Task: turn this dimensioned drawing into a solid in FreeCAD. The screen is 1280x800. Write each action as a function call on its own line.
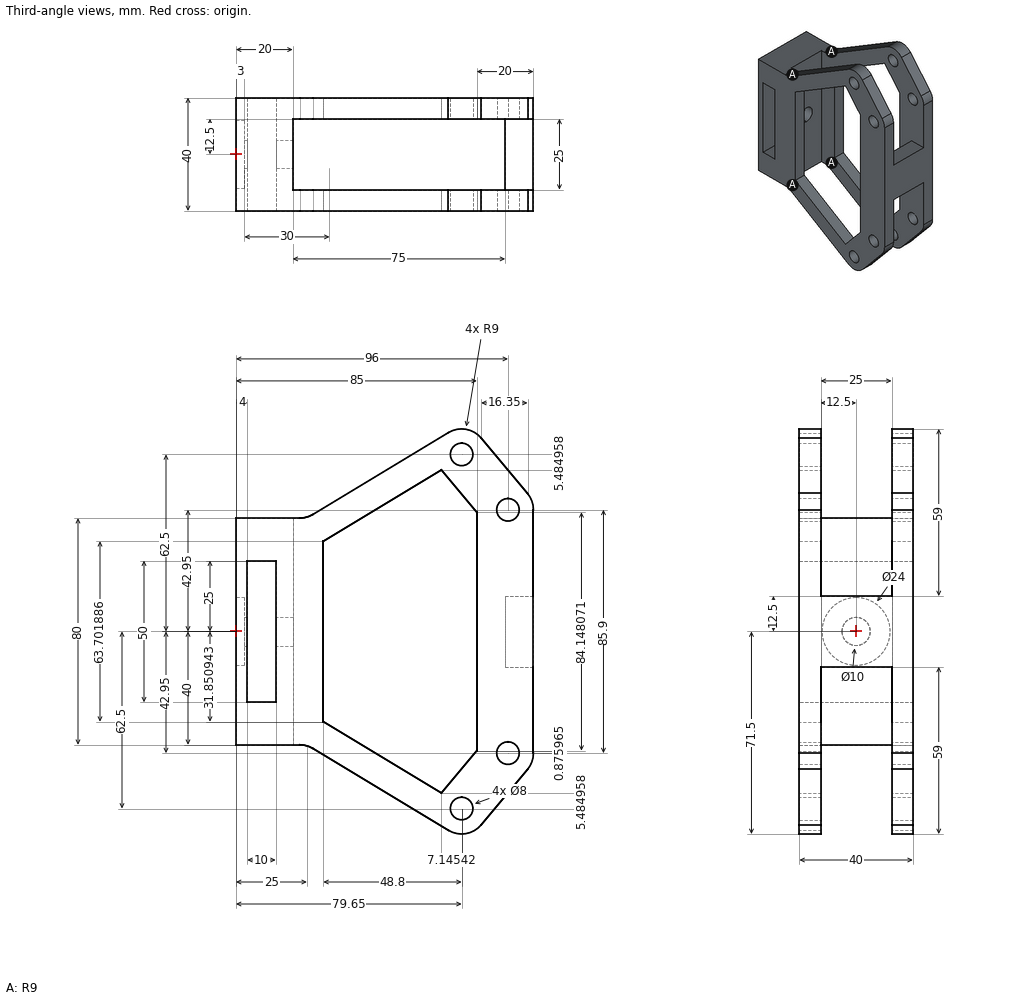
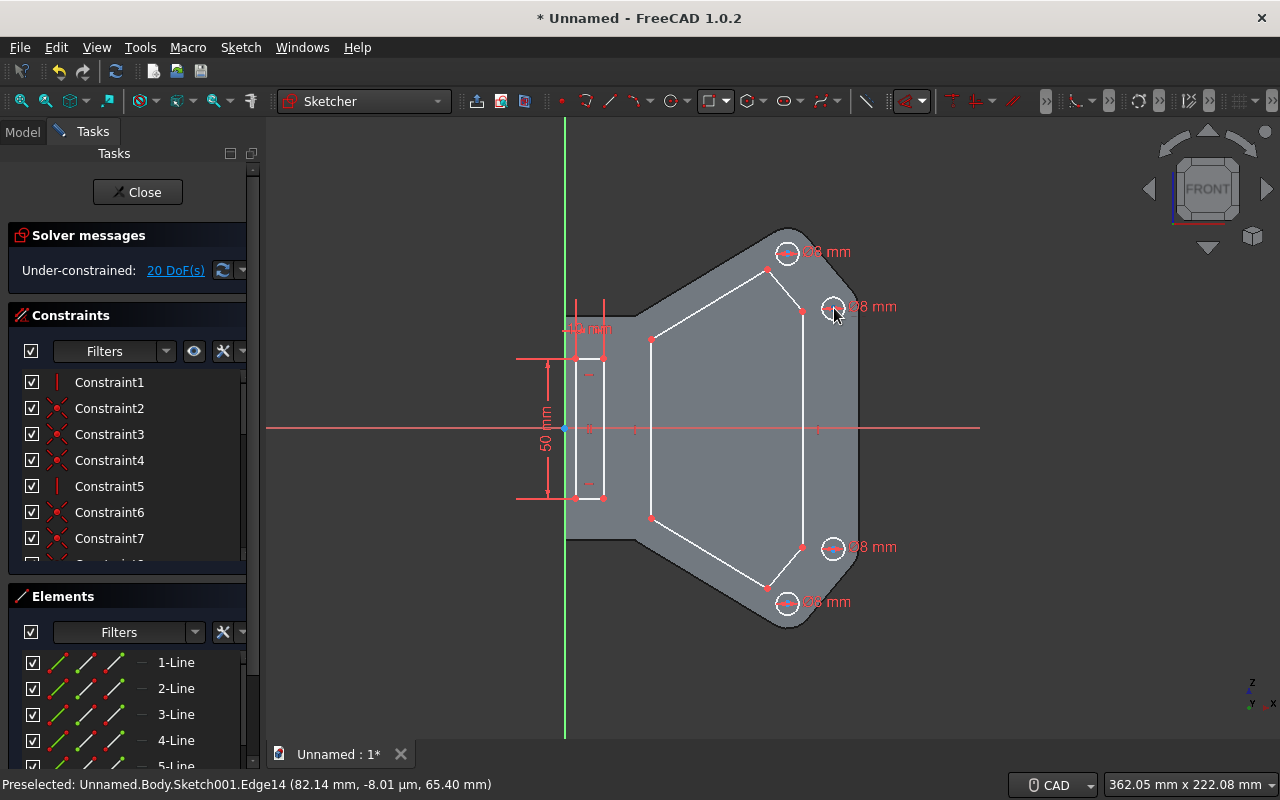
scroll(576, 359, up, 7)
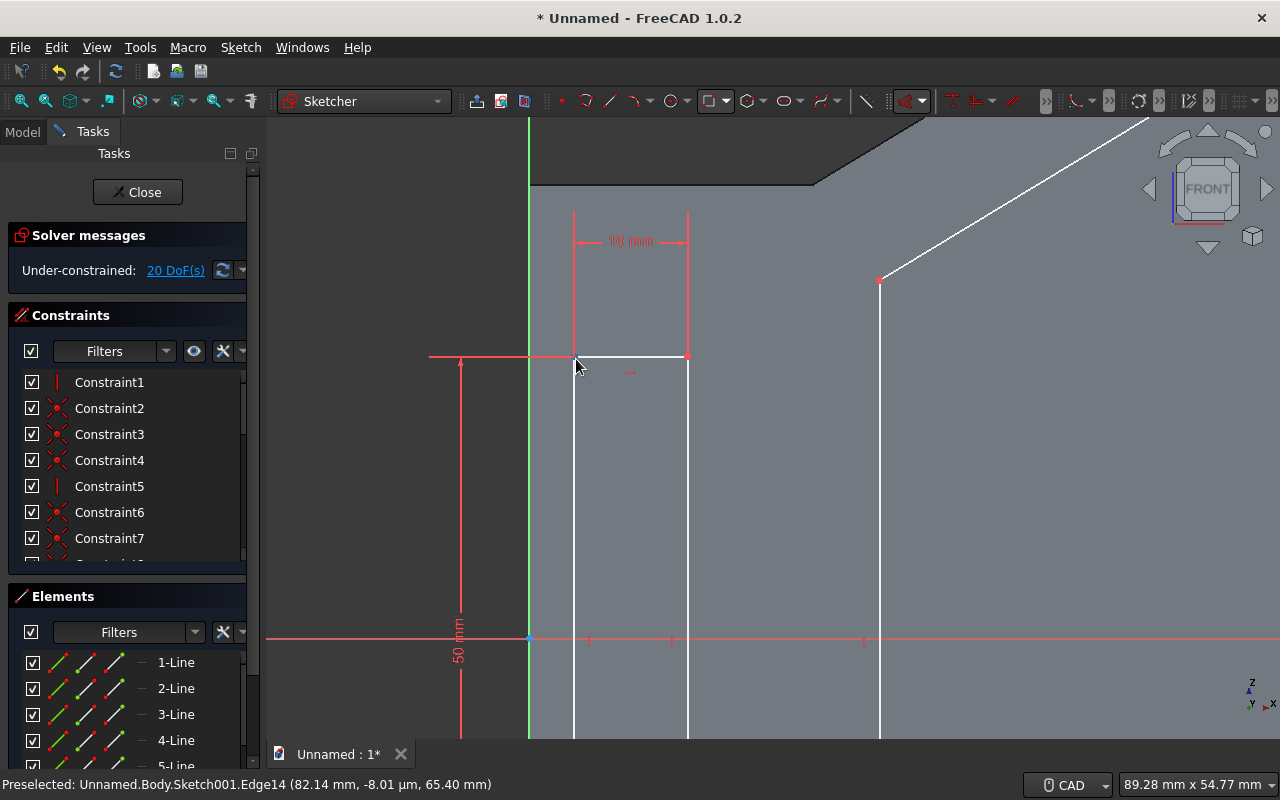
click(574, 357)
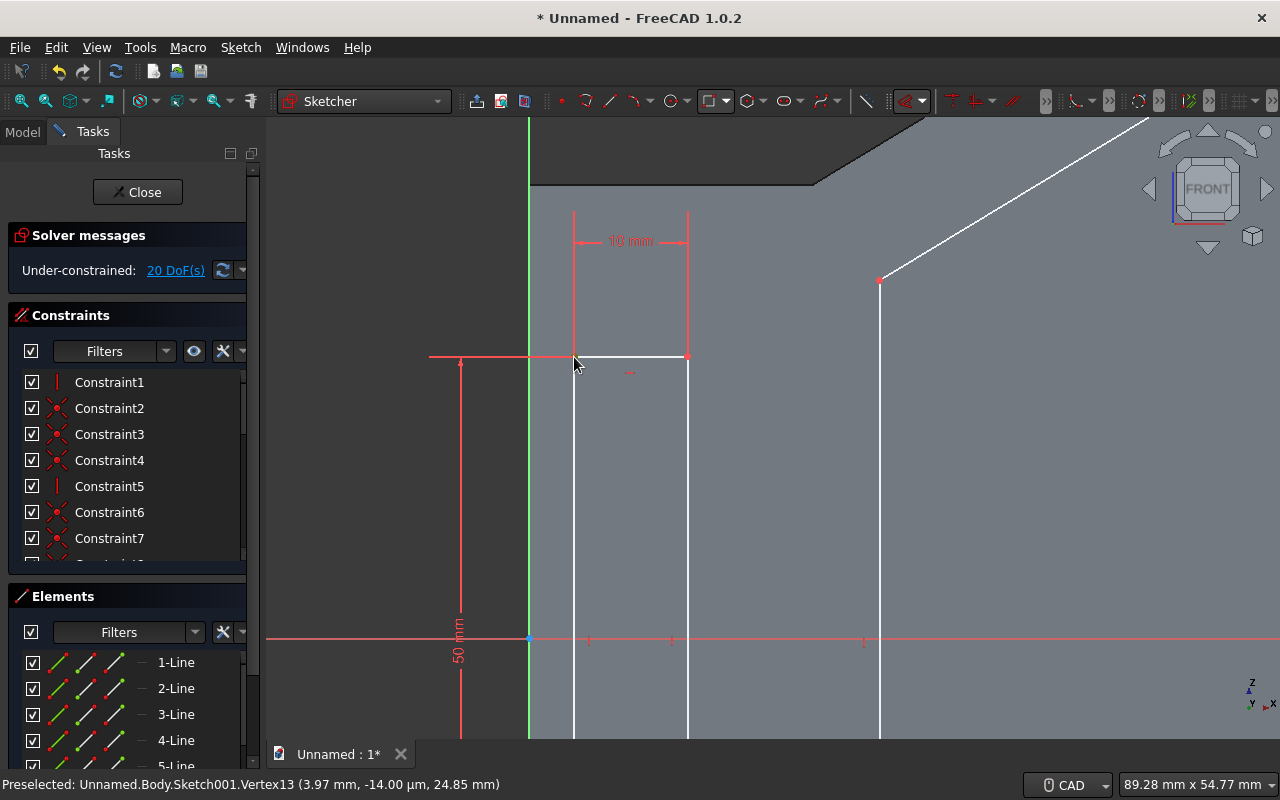
key(l)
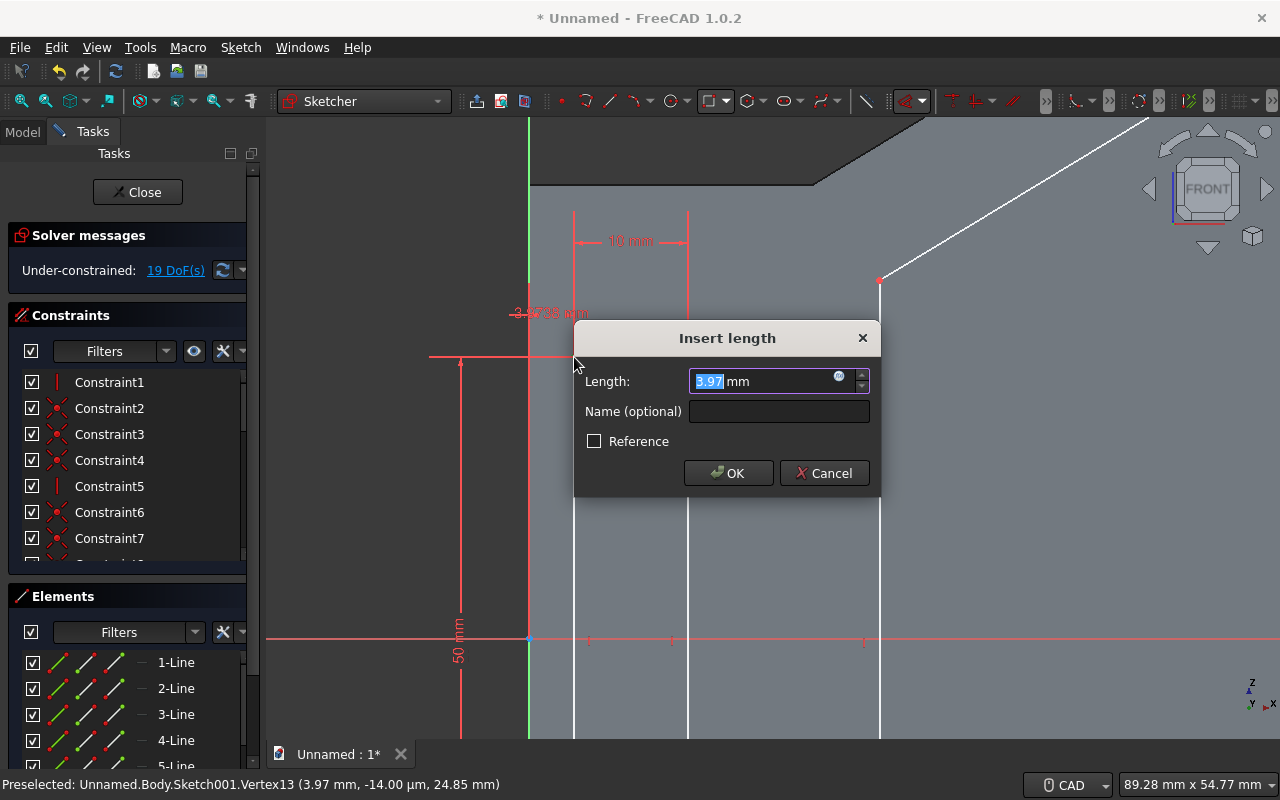
text(4)
key(Return)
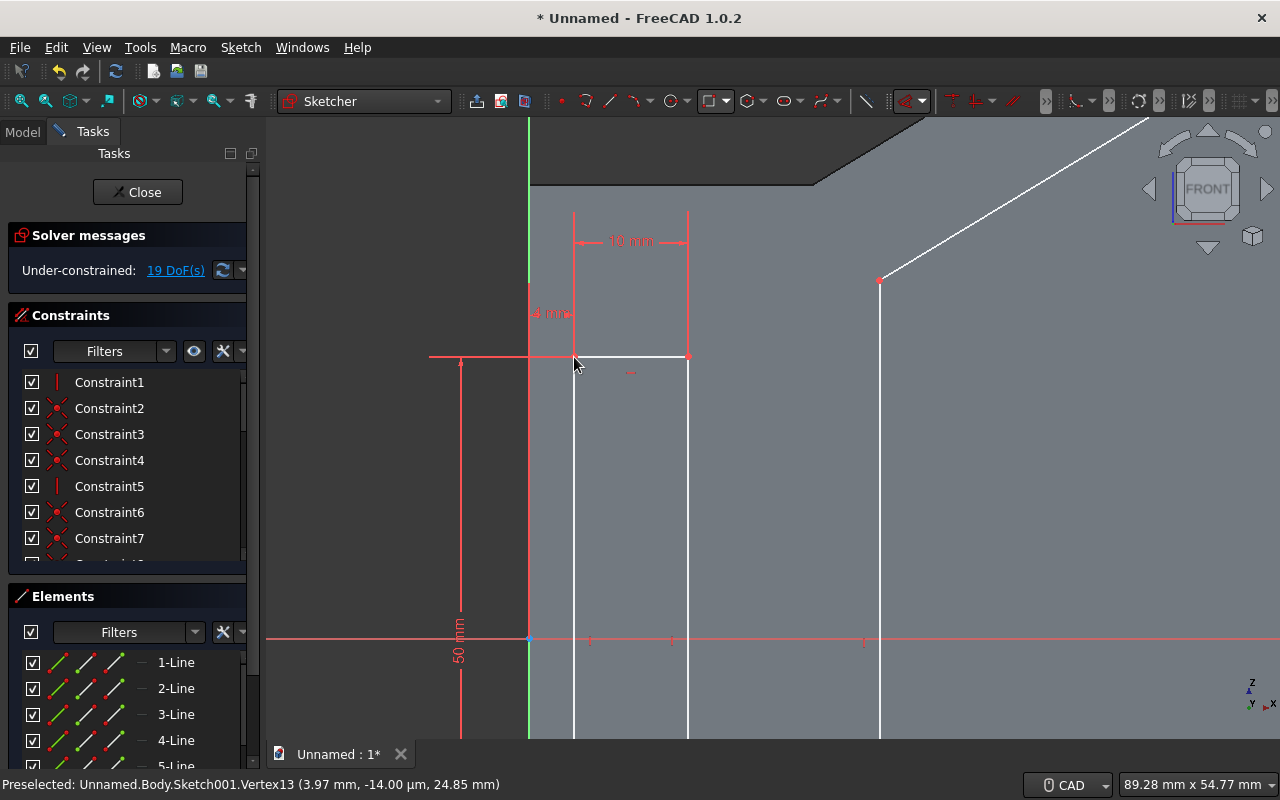
scroll(576, 359, down, 7)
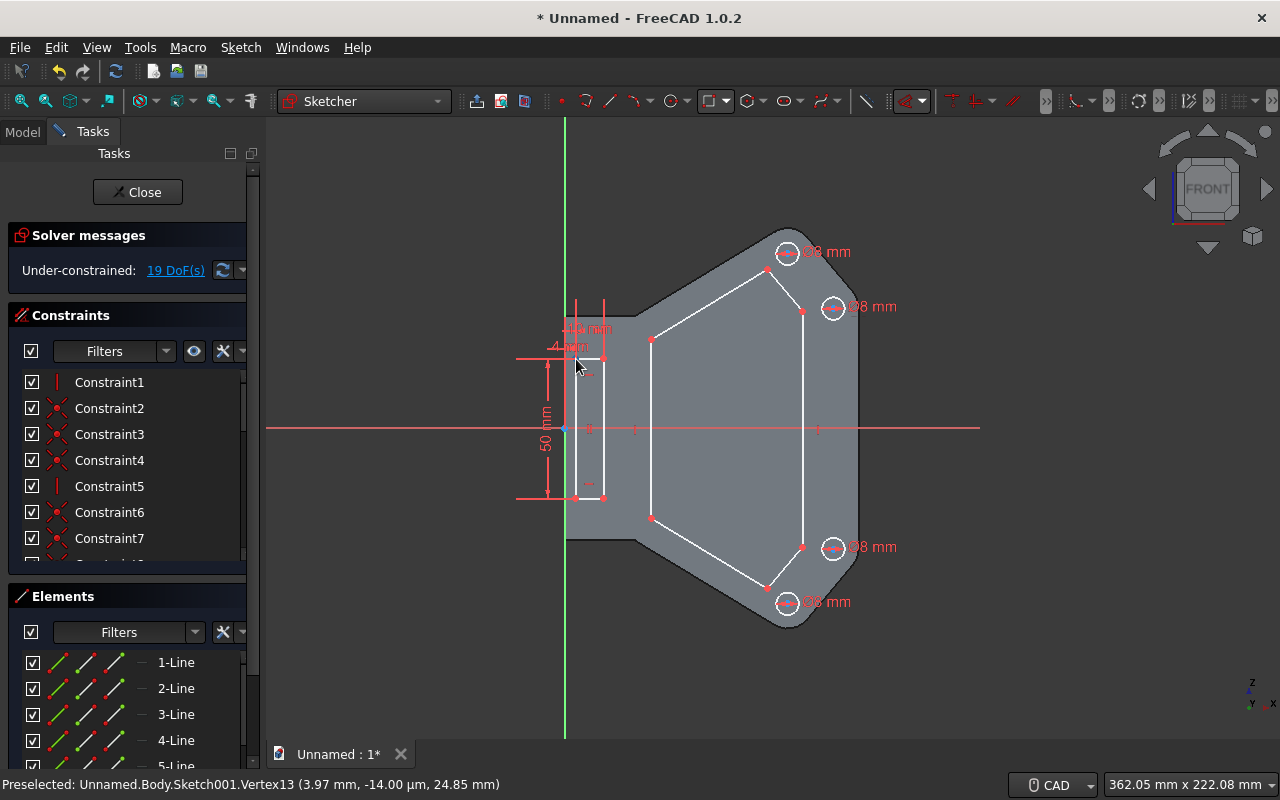
click(833, 549)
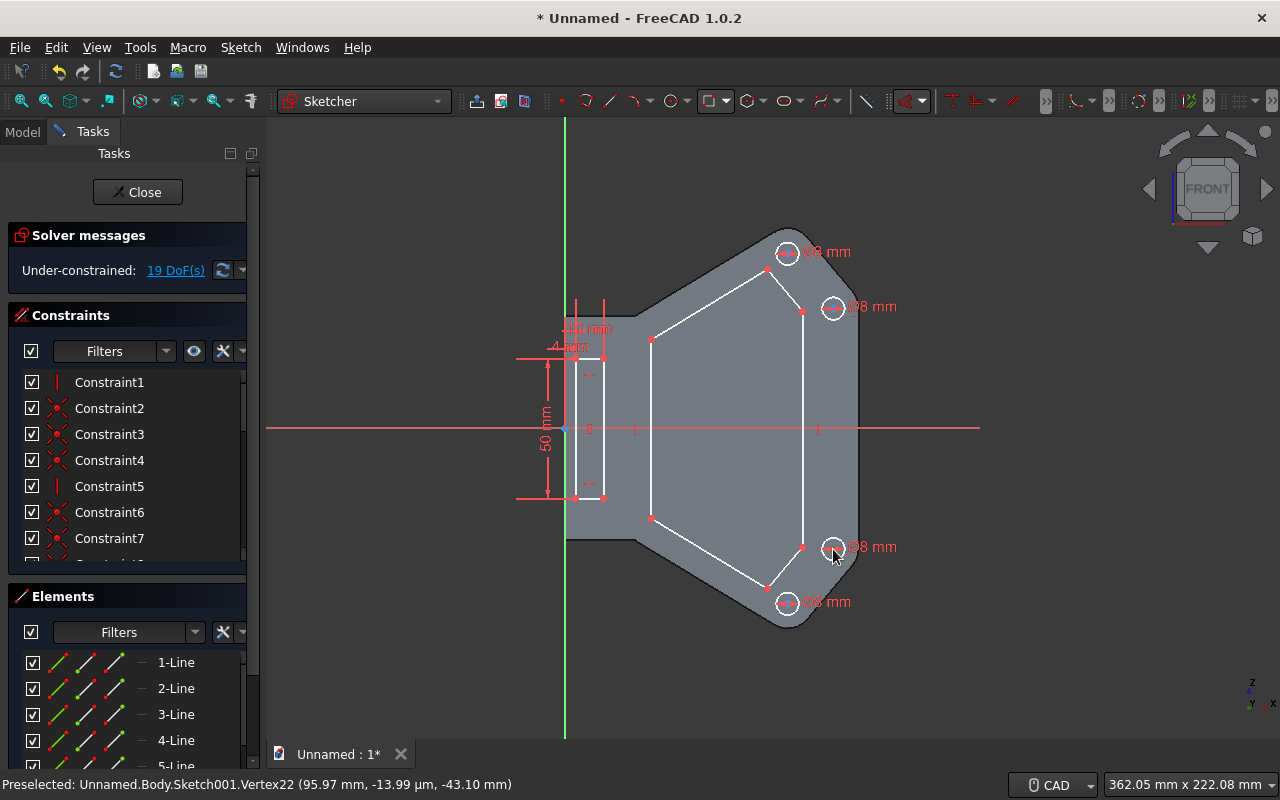
key(l)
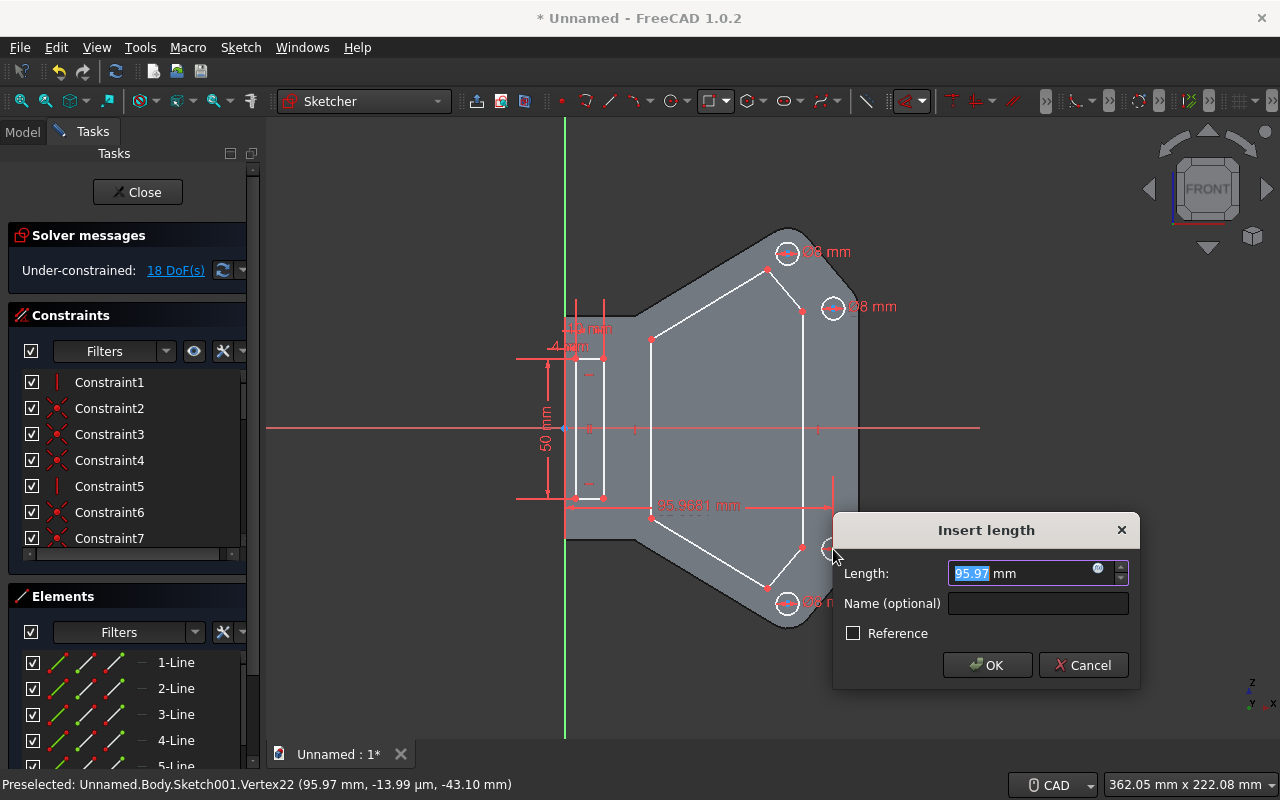
text(96)
key(Return)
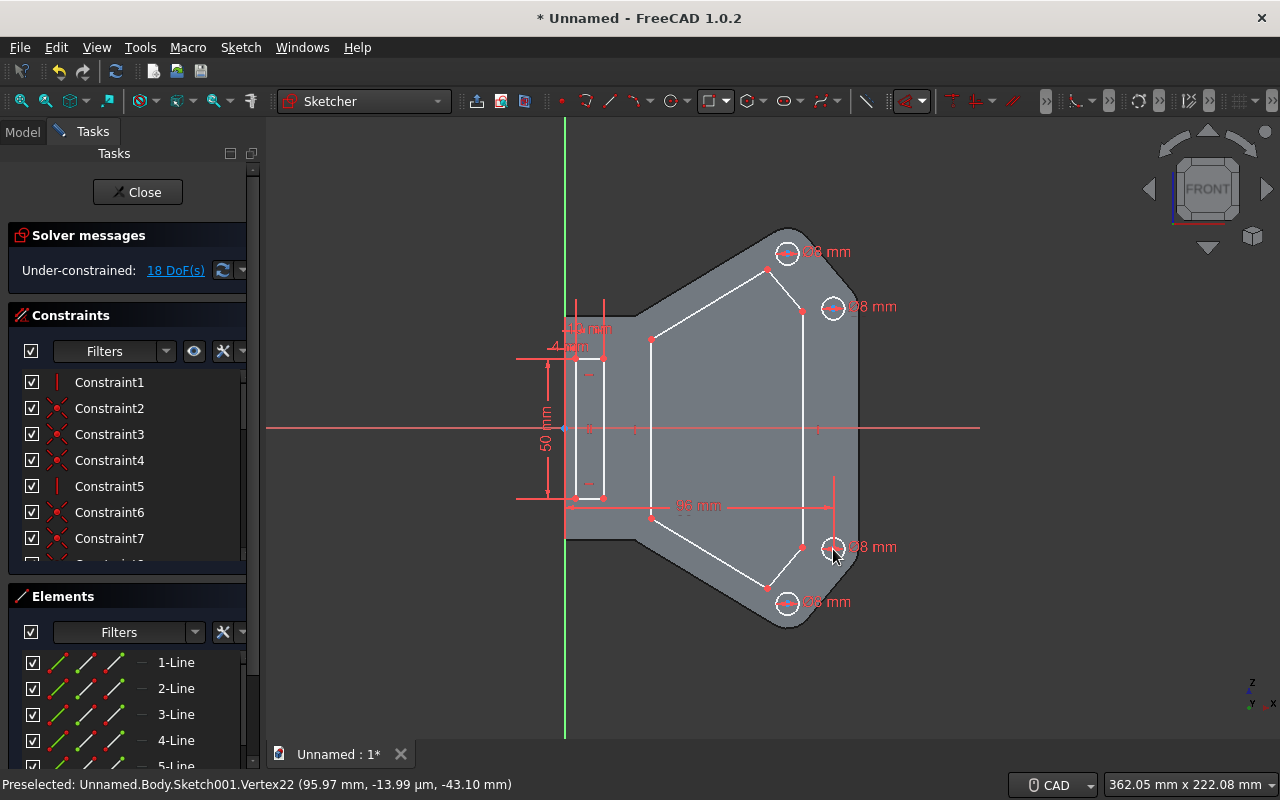
click(833, 309)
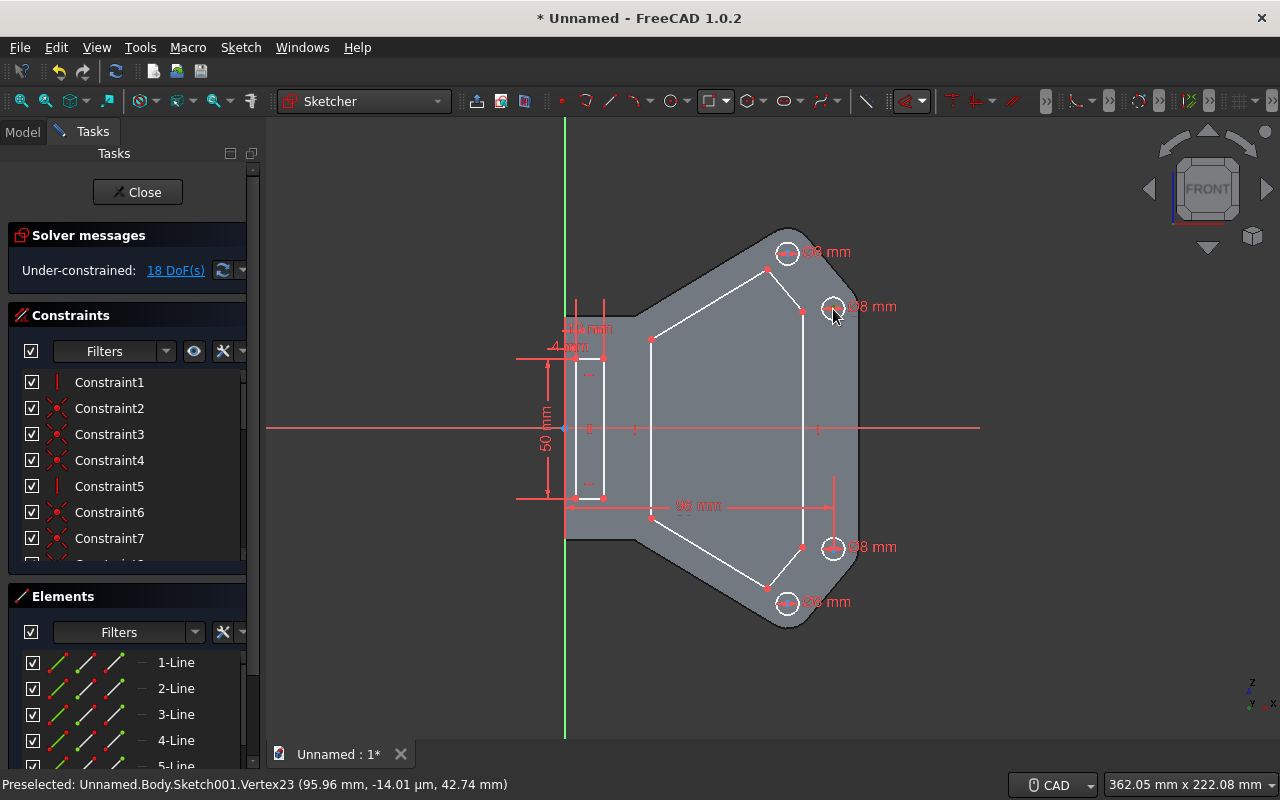
click(924, 102)